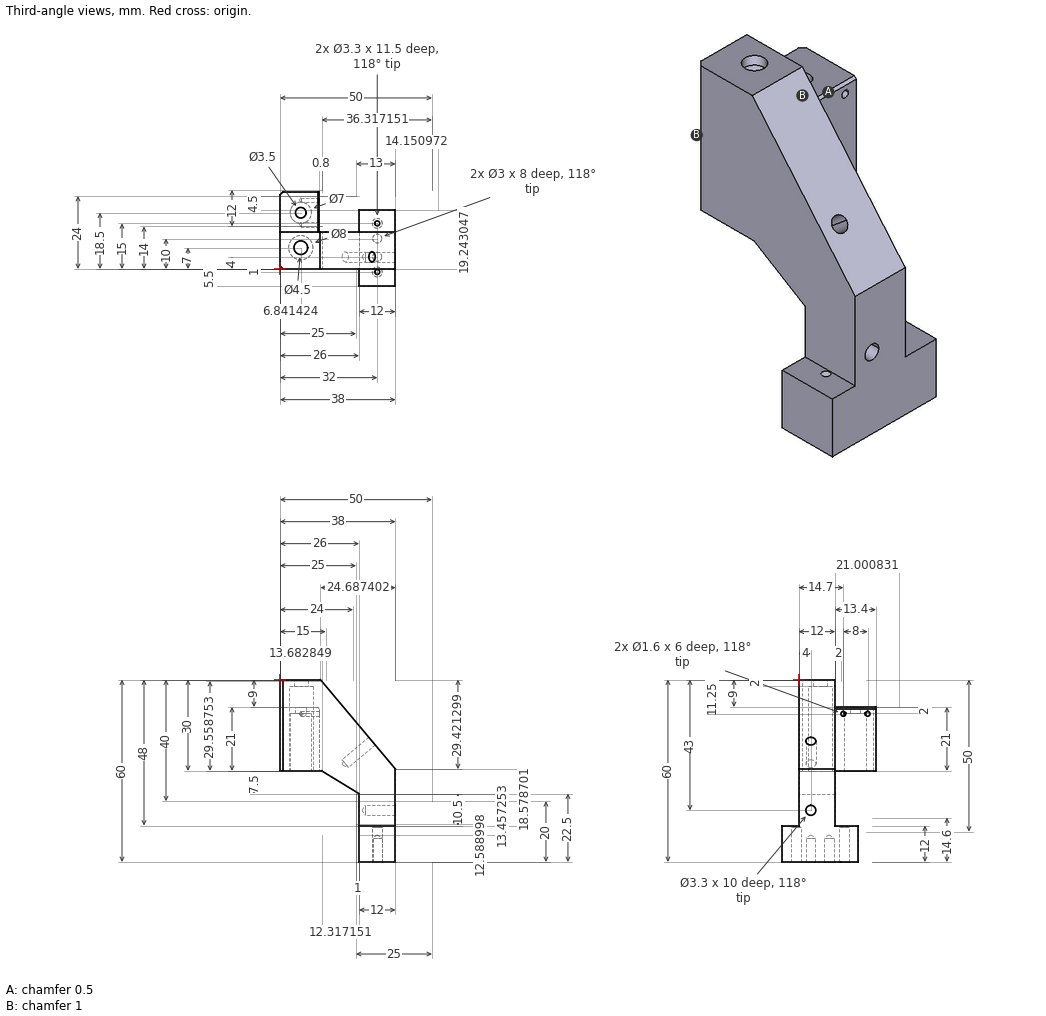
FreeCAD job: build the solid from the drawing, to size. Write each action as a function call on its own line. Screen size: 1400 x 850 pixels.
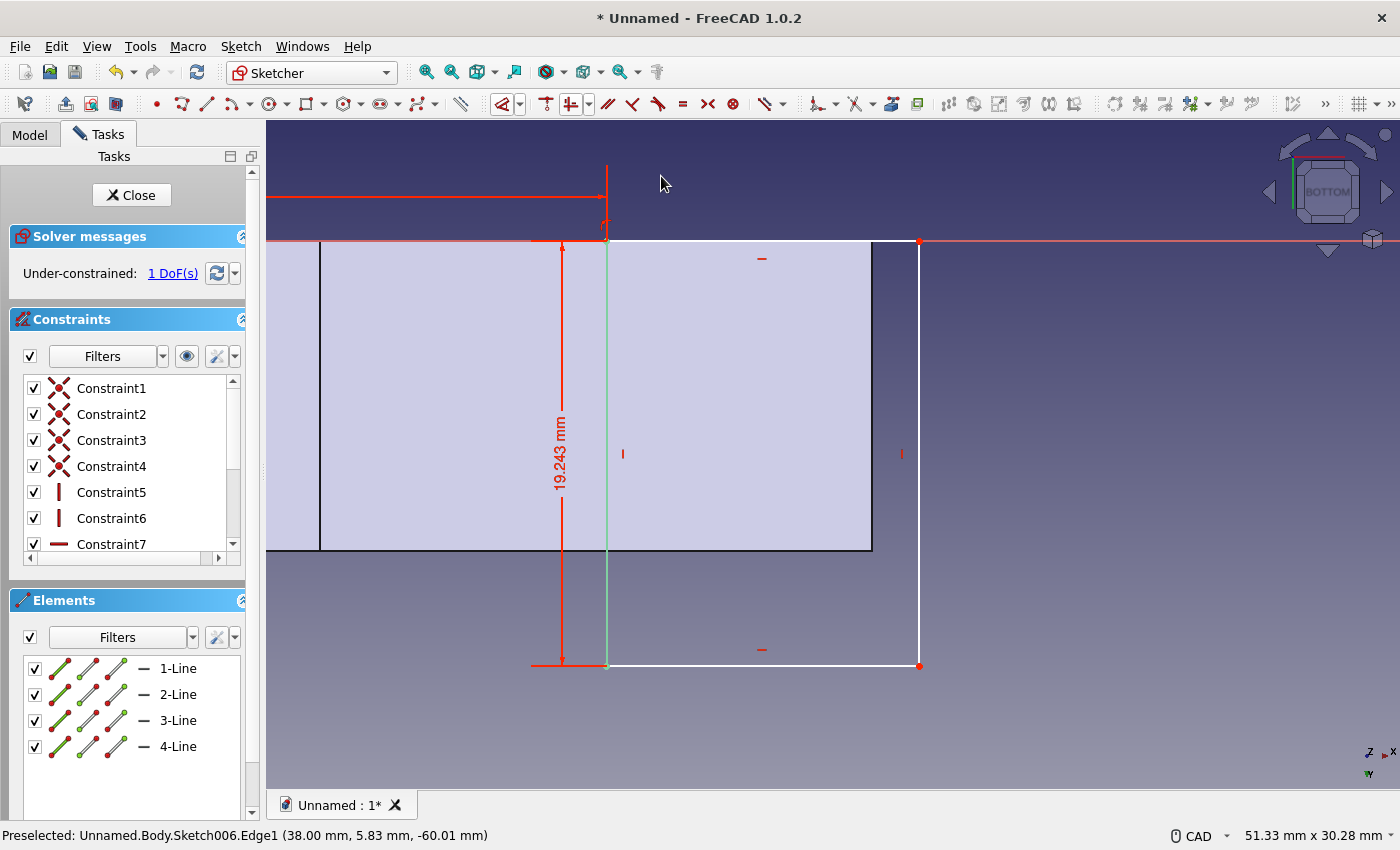
click(700, 666)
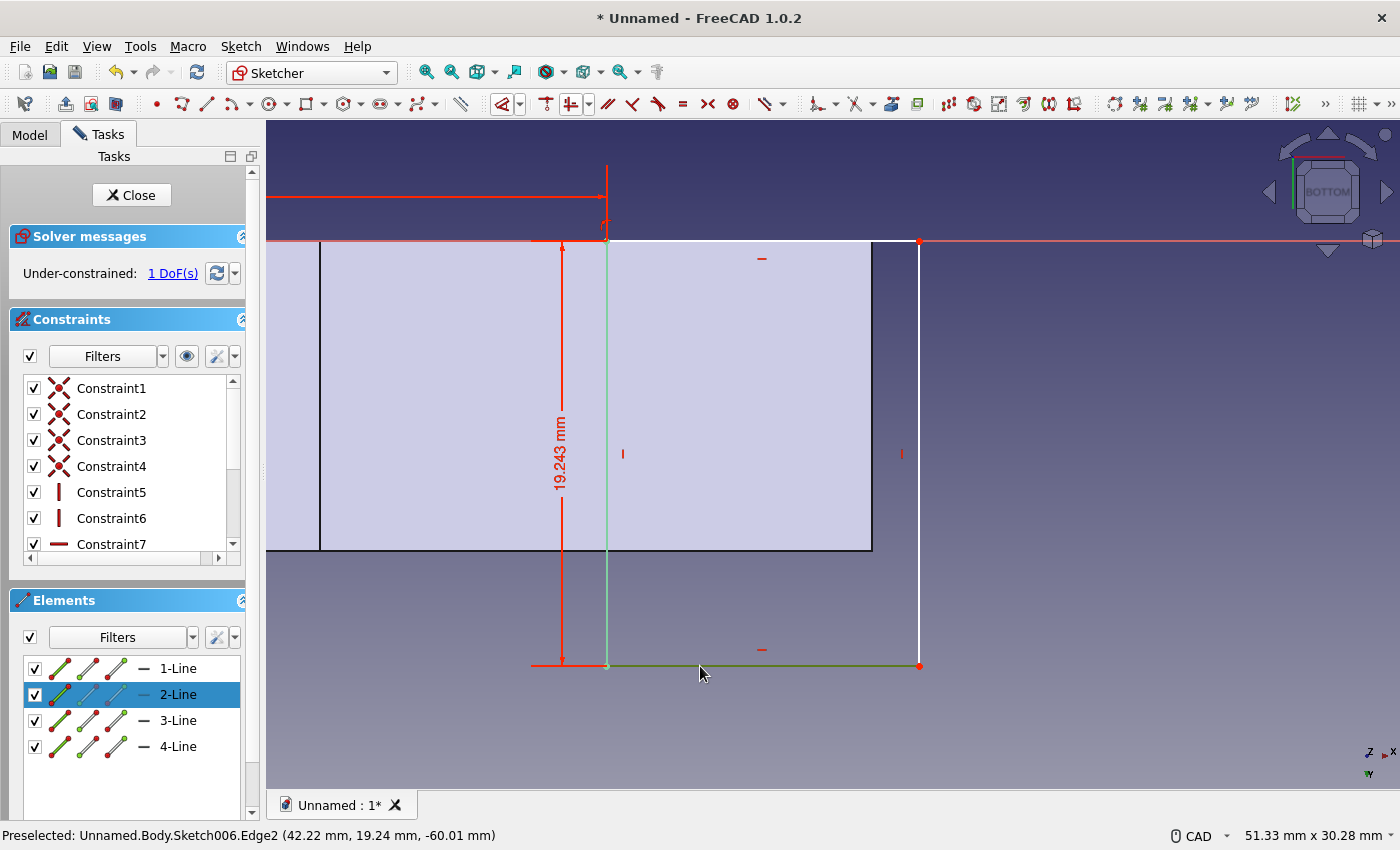
key(l)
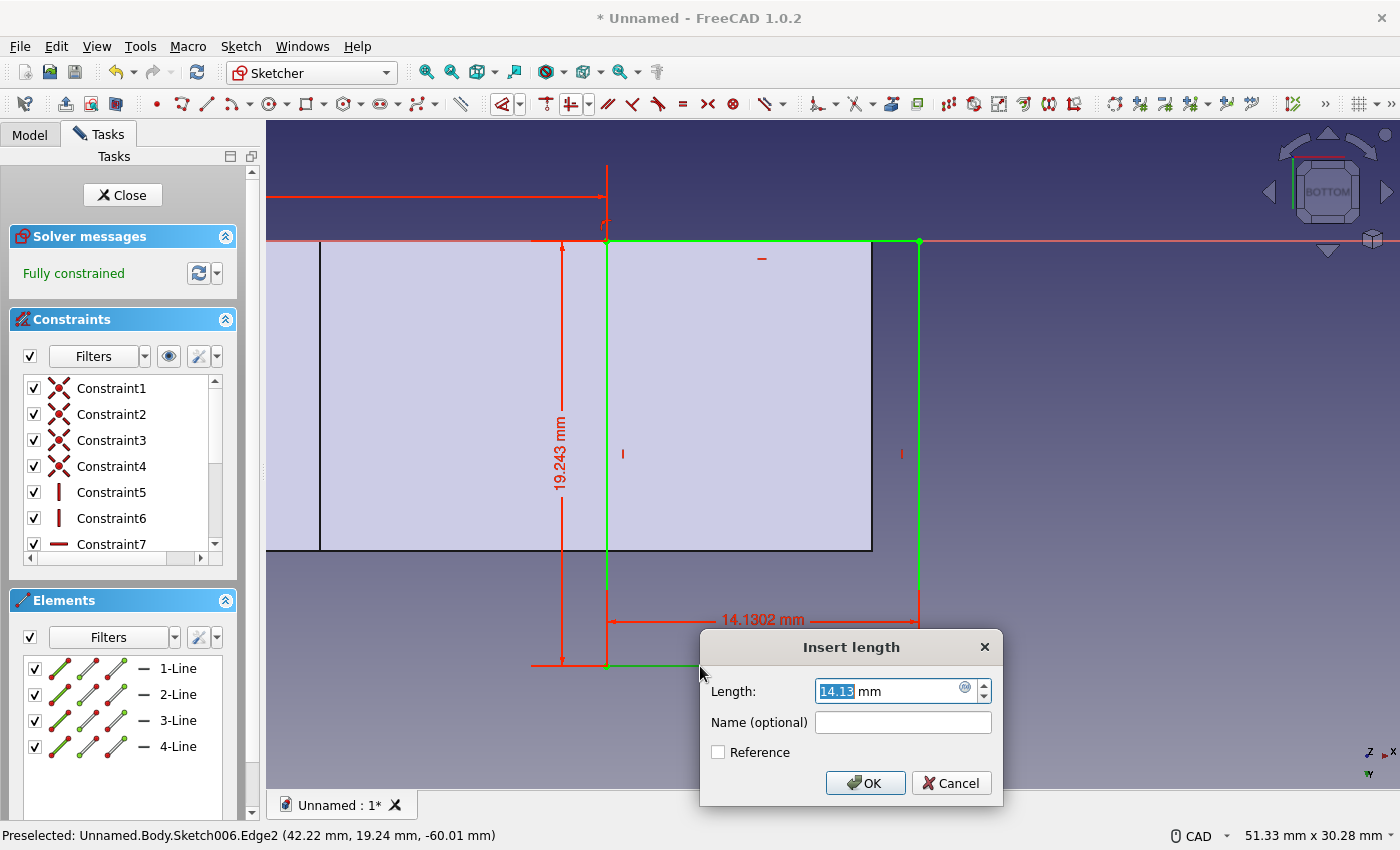
text(14.150972)
key(Return)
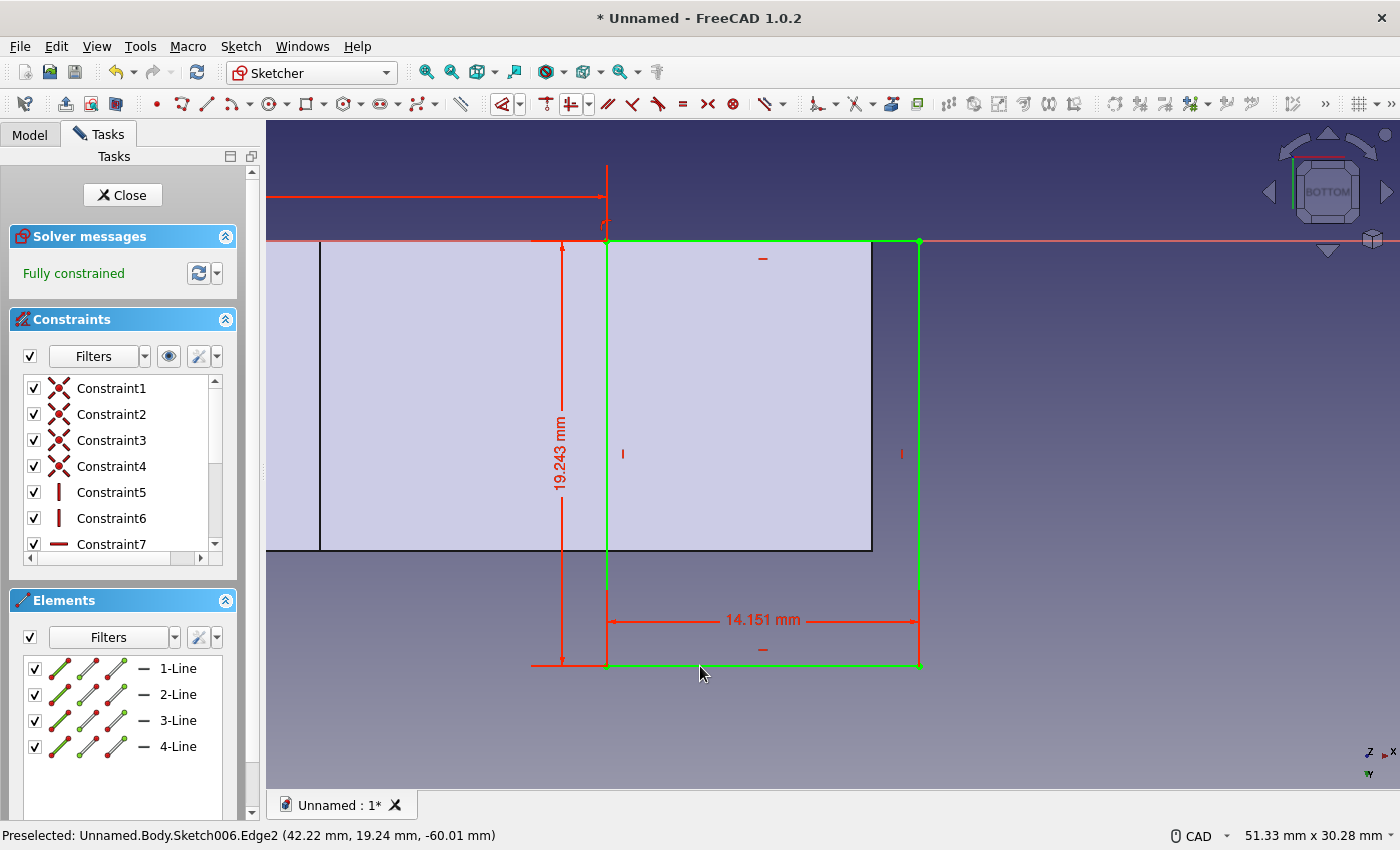
click(123, 195)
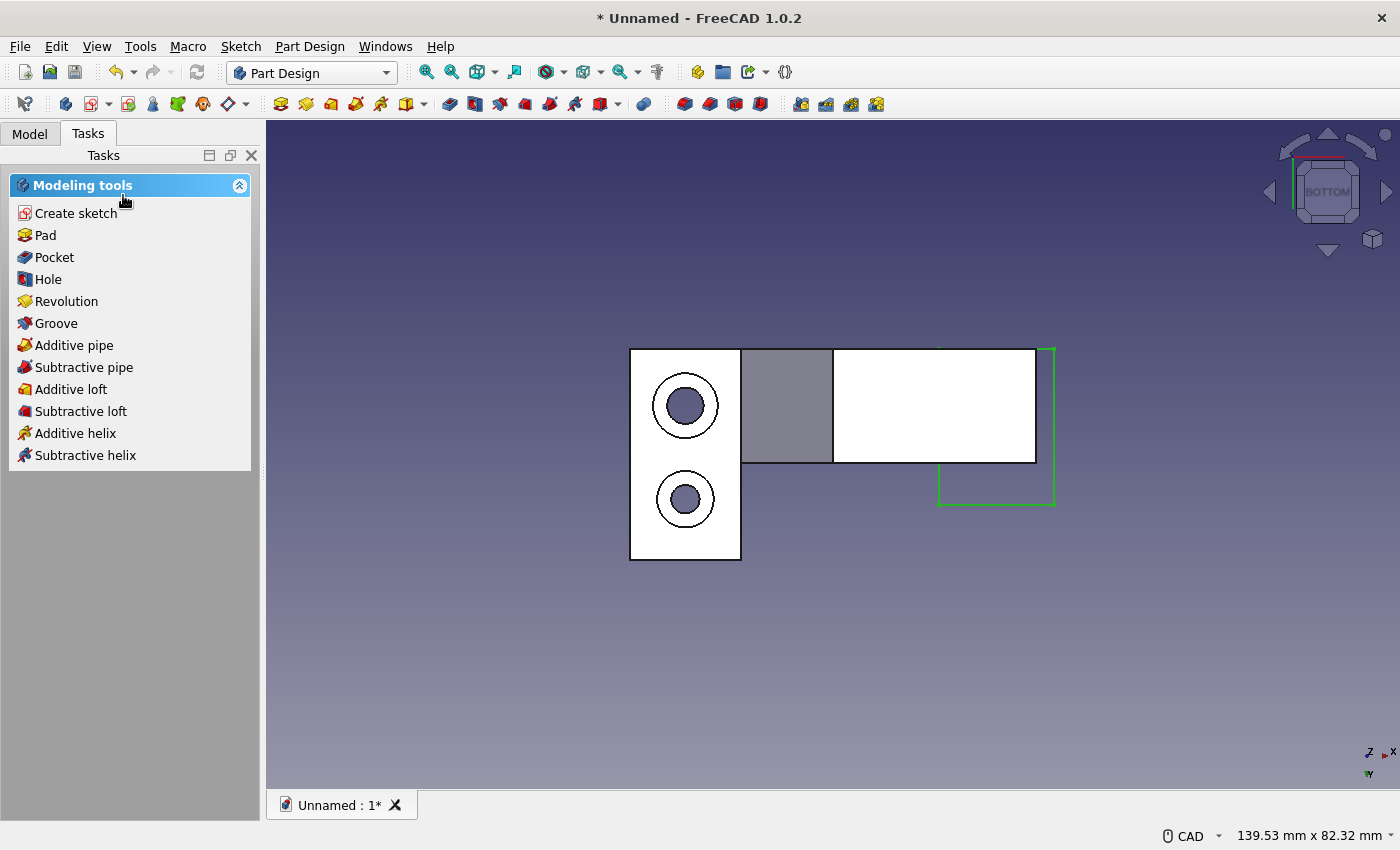
click(450, 104)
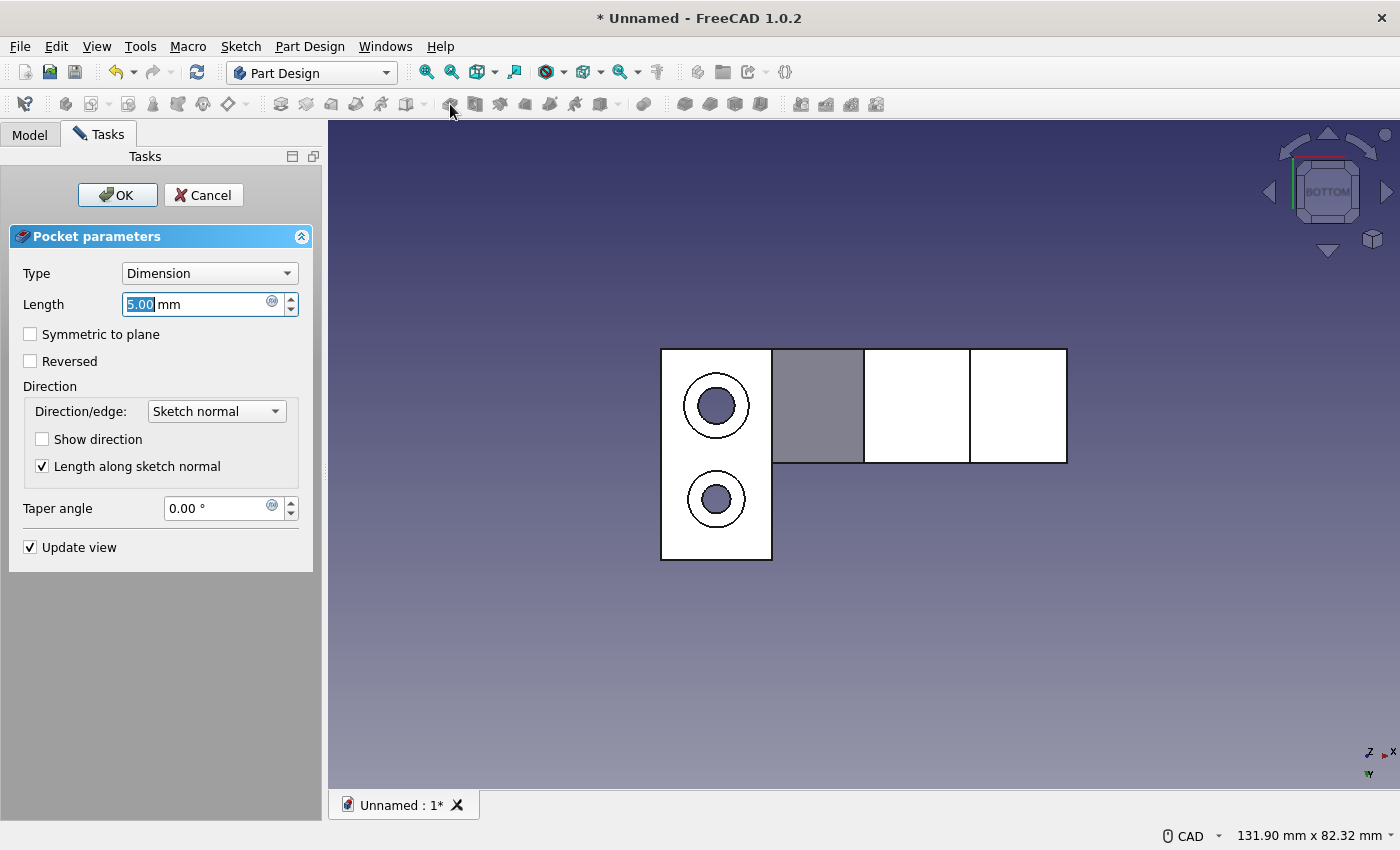
text(60)
key(Tab)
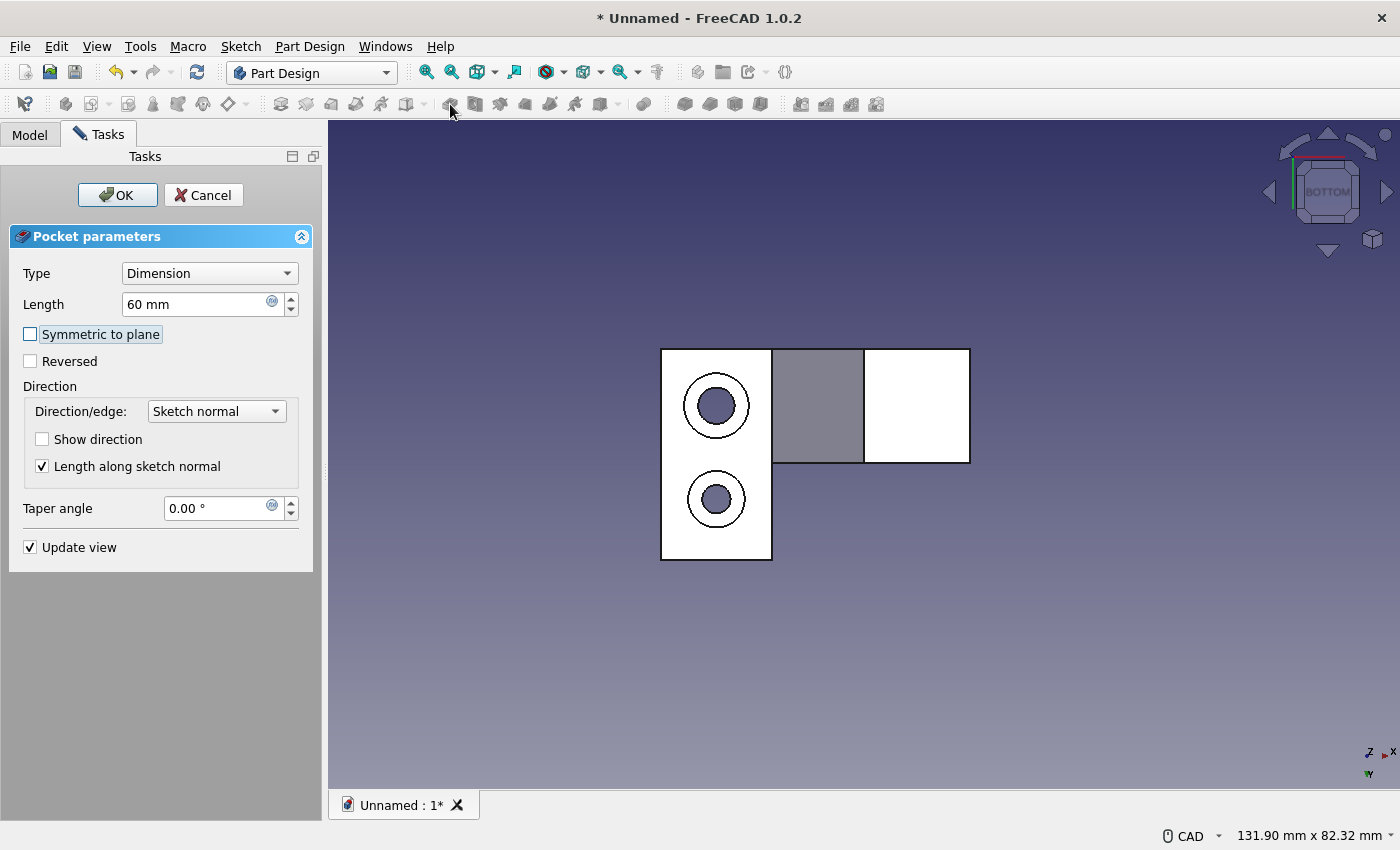
click(118, 195)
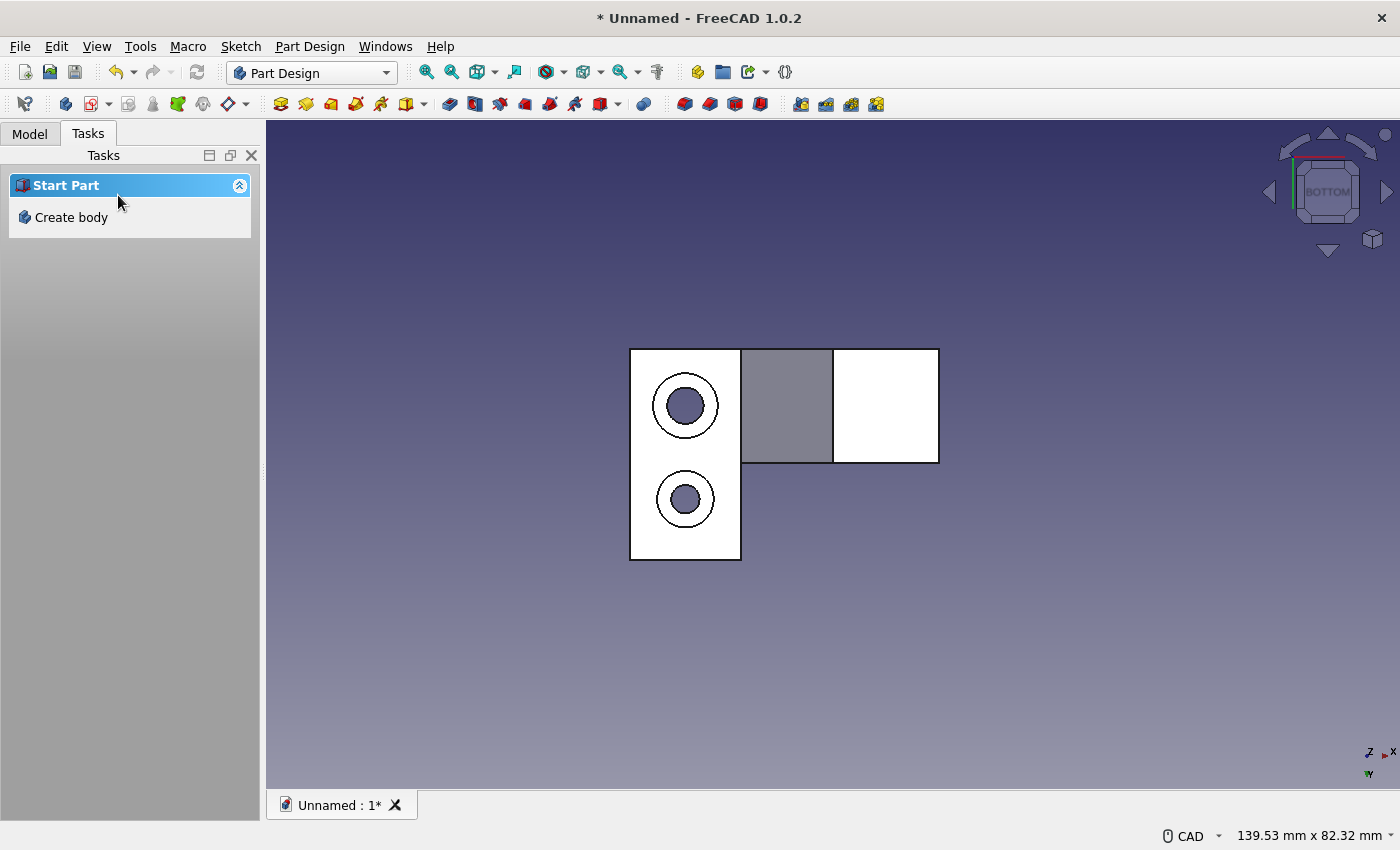
click(427, 72)